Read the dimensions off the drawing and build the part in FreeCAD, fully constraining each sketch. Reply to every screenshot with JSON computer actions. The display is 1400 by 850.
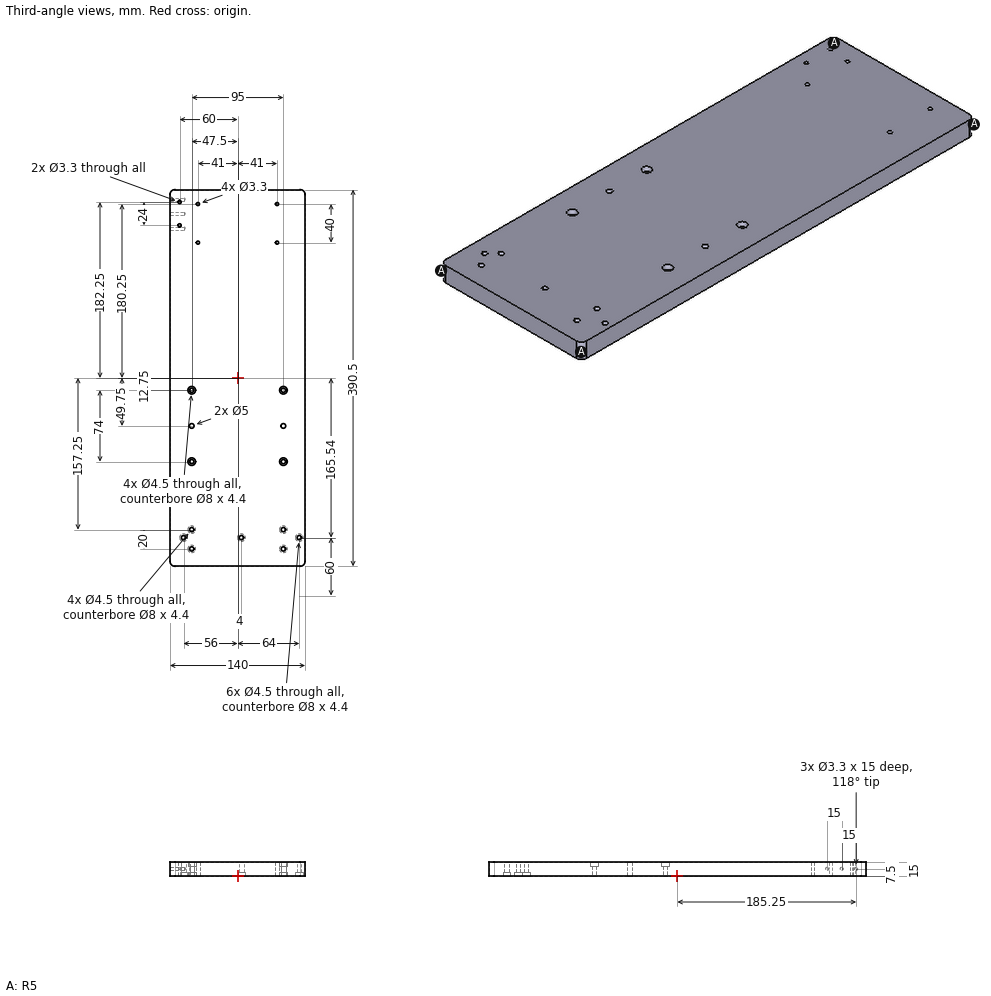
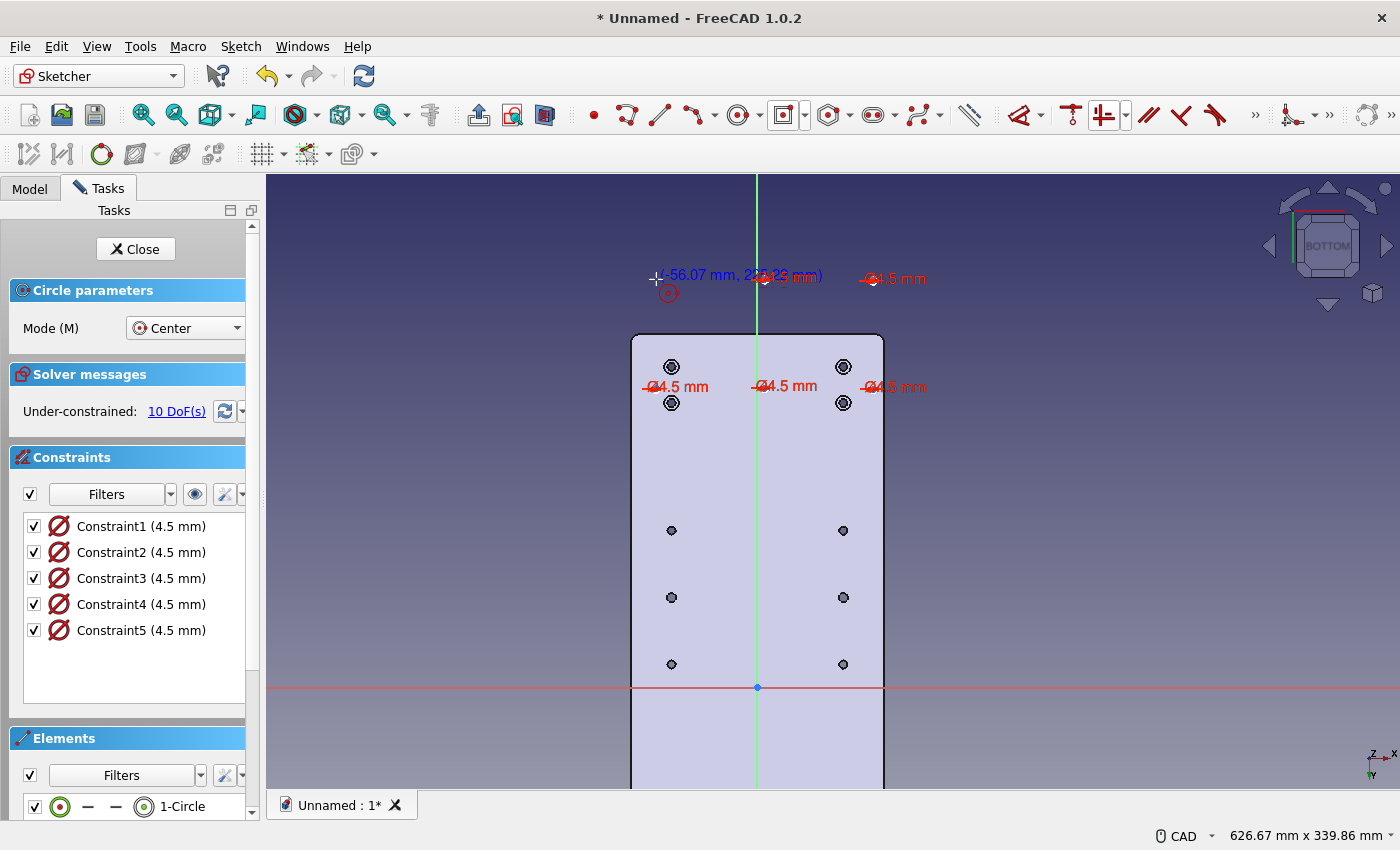
{"action": "left_click", "coordinate": [656, 279]}
{"action": "mouse_move", "coordinate": [659, 277]}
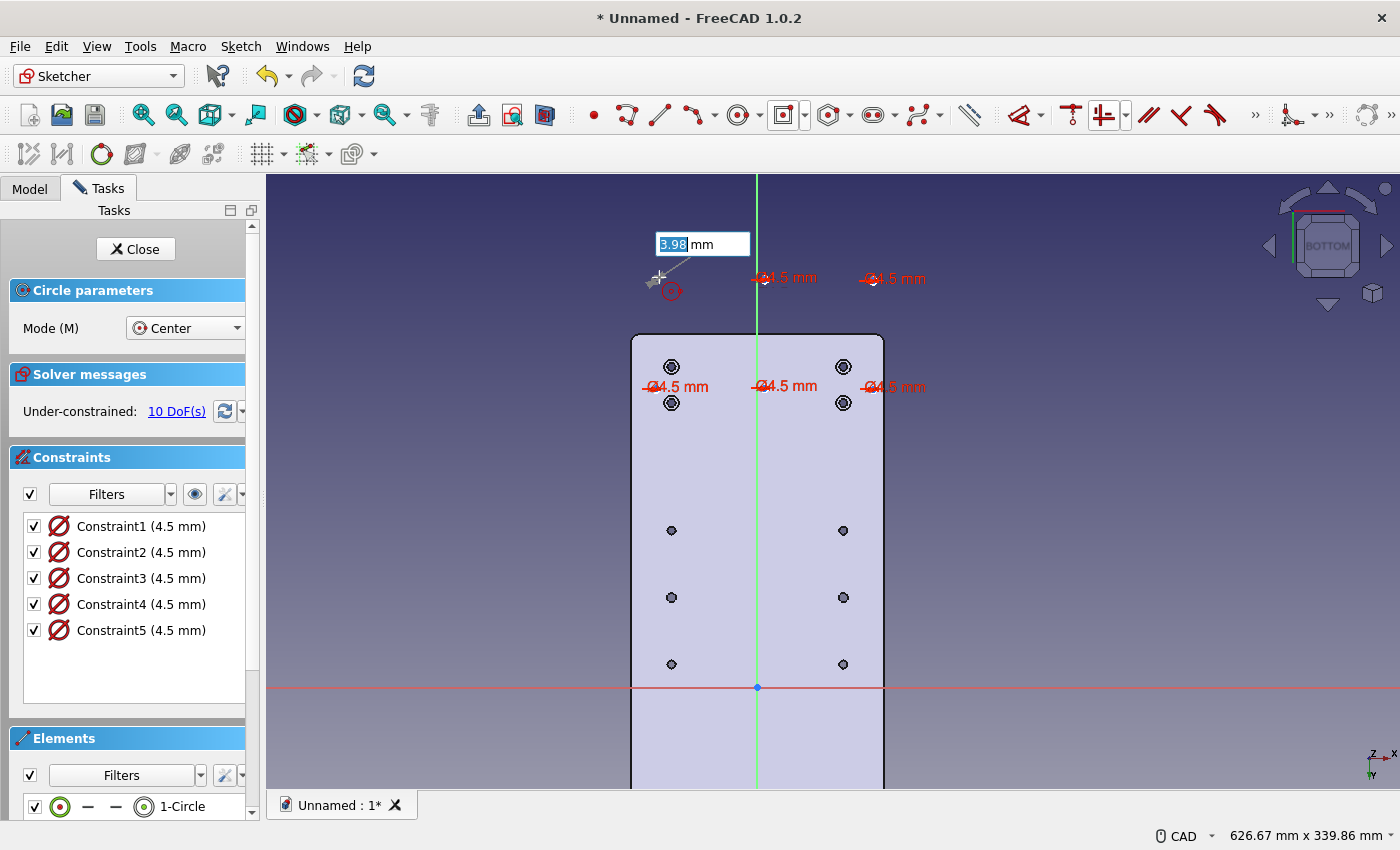
{"action": "type", "text": "4.5"}
{"action": "key", "text": "Return"}
{"action": "key", "text": "Escape"}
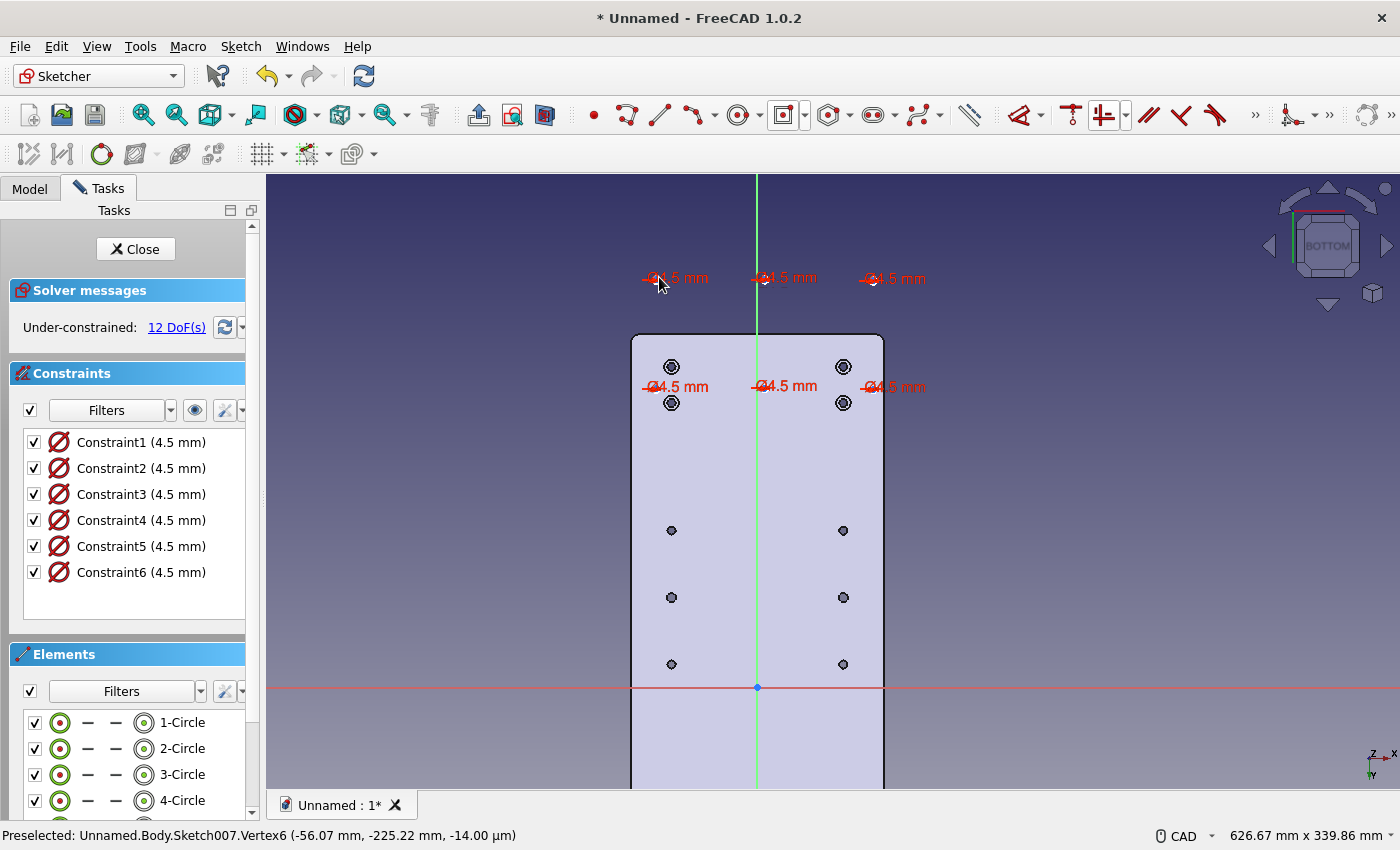
{"action": "left_click", "coordinate": [873, 389]}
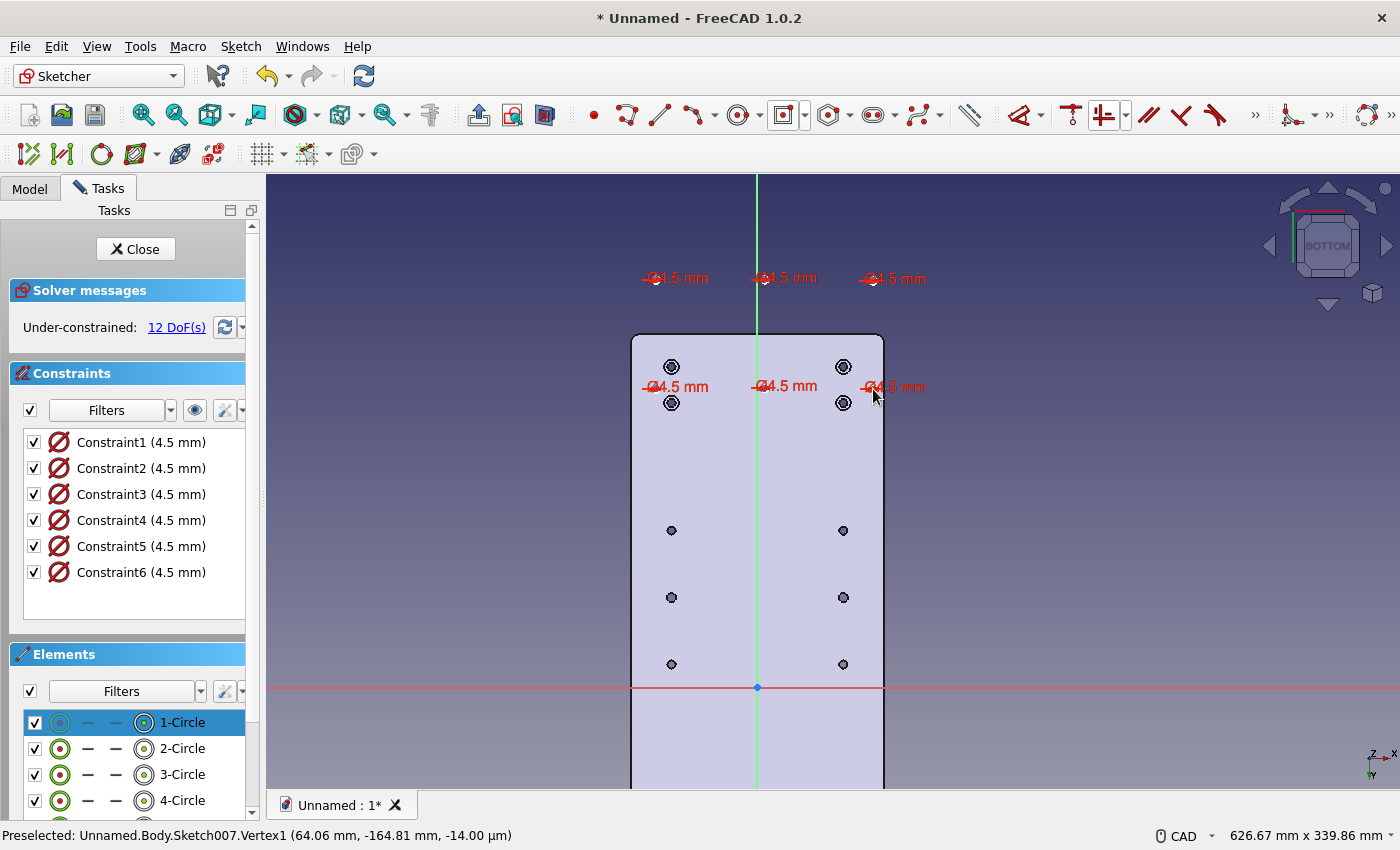
{"action": "left_click", "coordinate": [765, 388]}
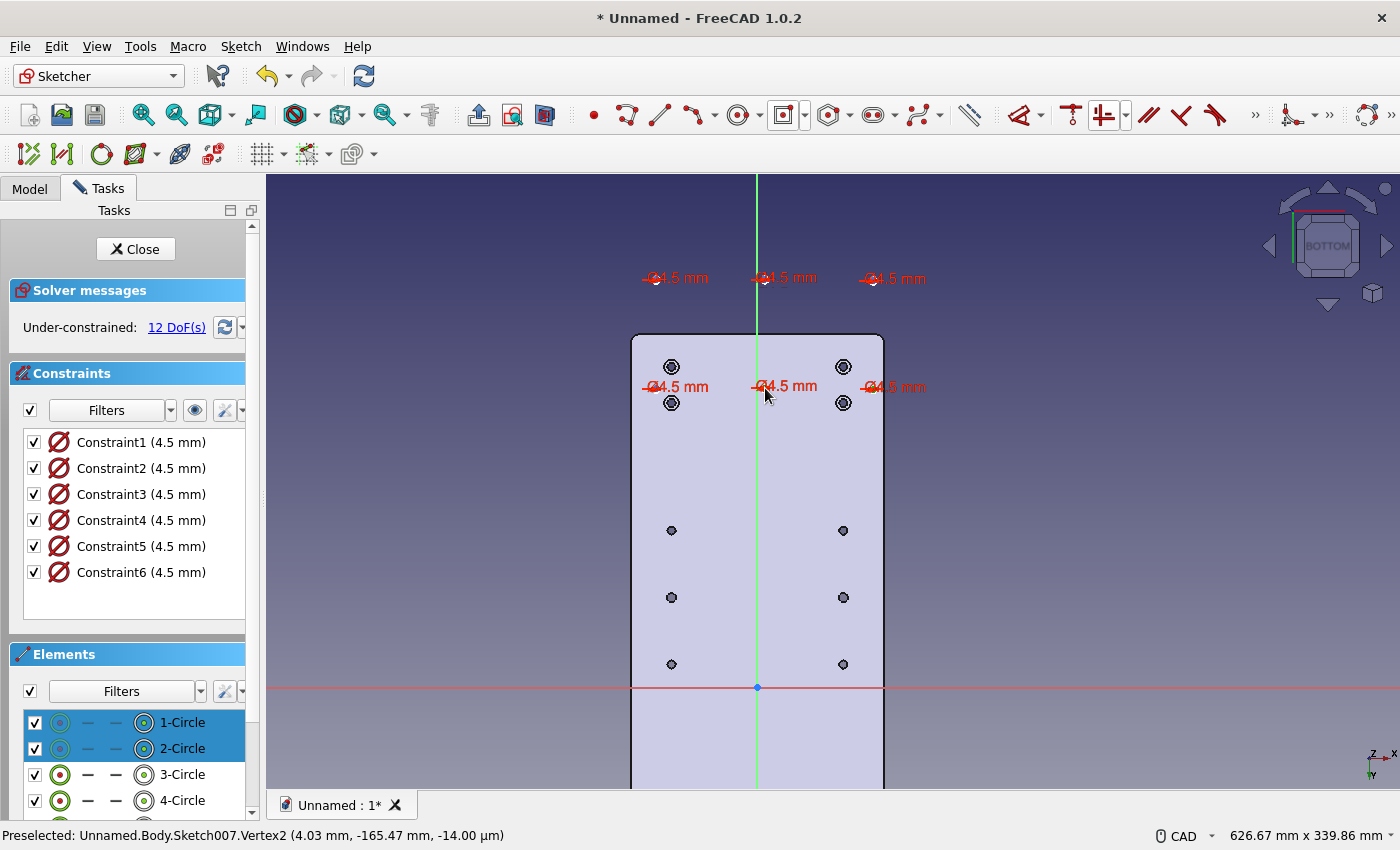
{"action": "key", "text": "h"}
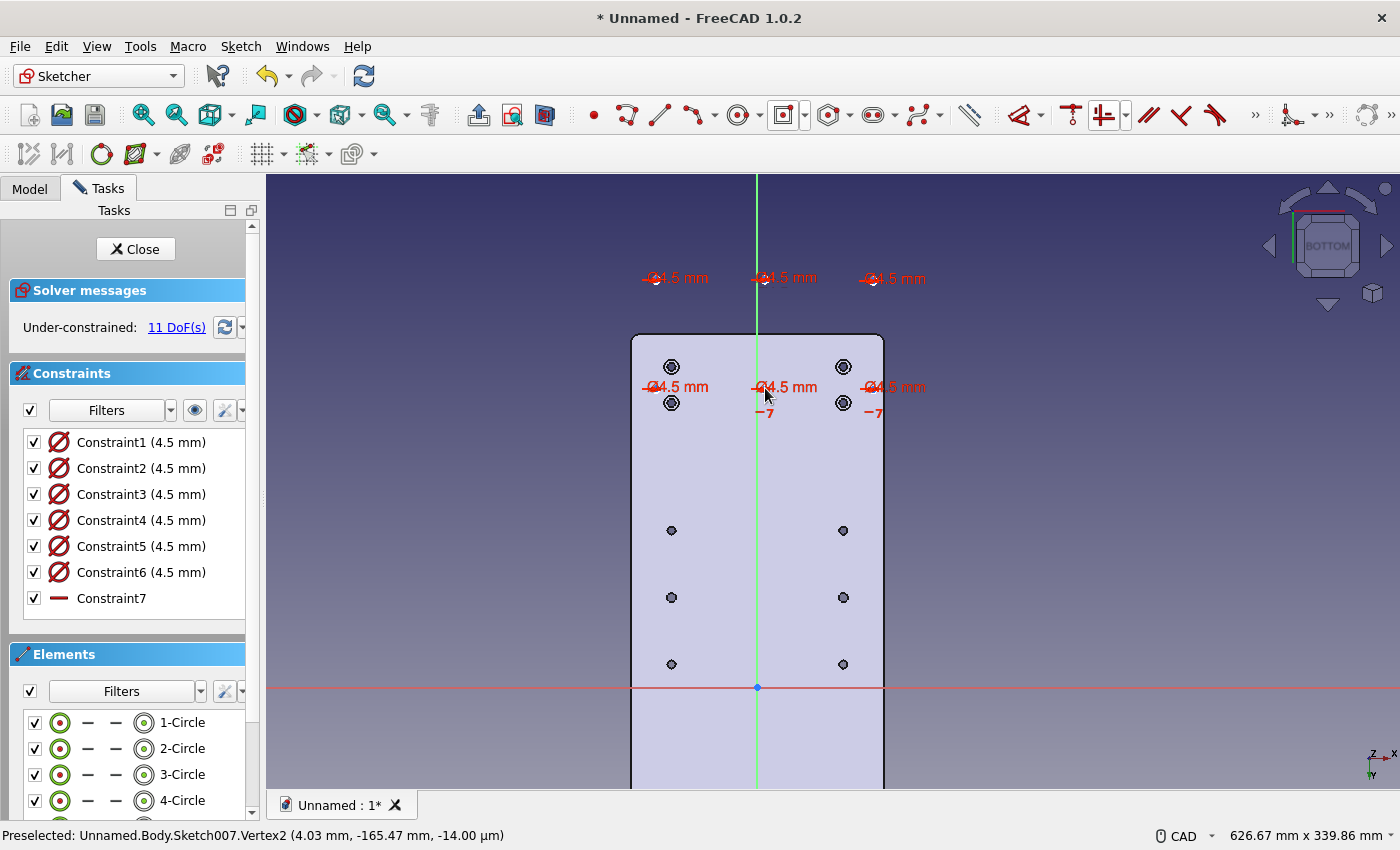
{"action": "left_click", "coordinate": [873, 389]}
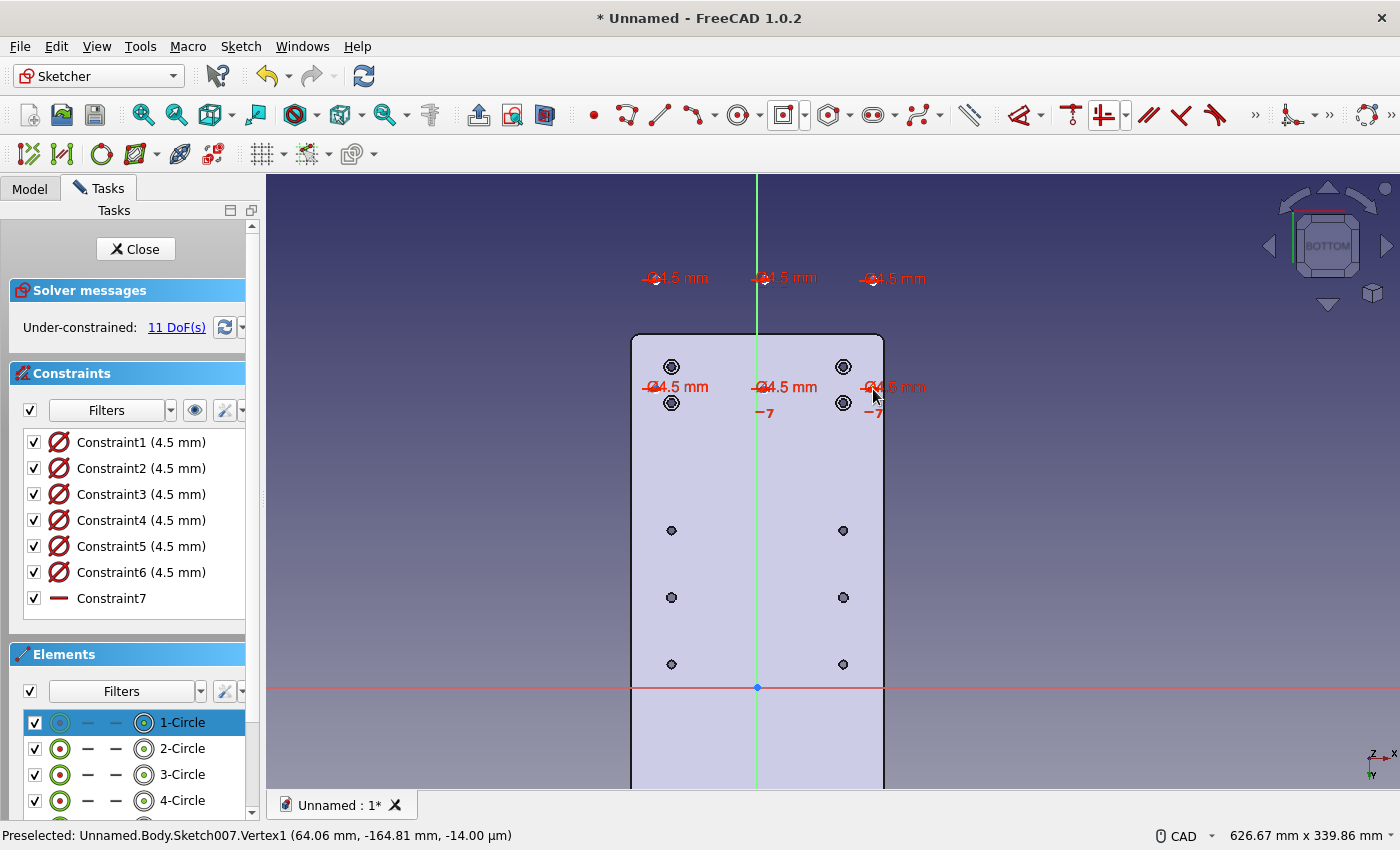
{"action": "left_click", "coordinate": [873, 281]}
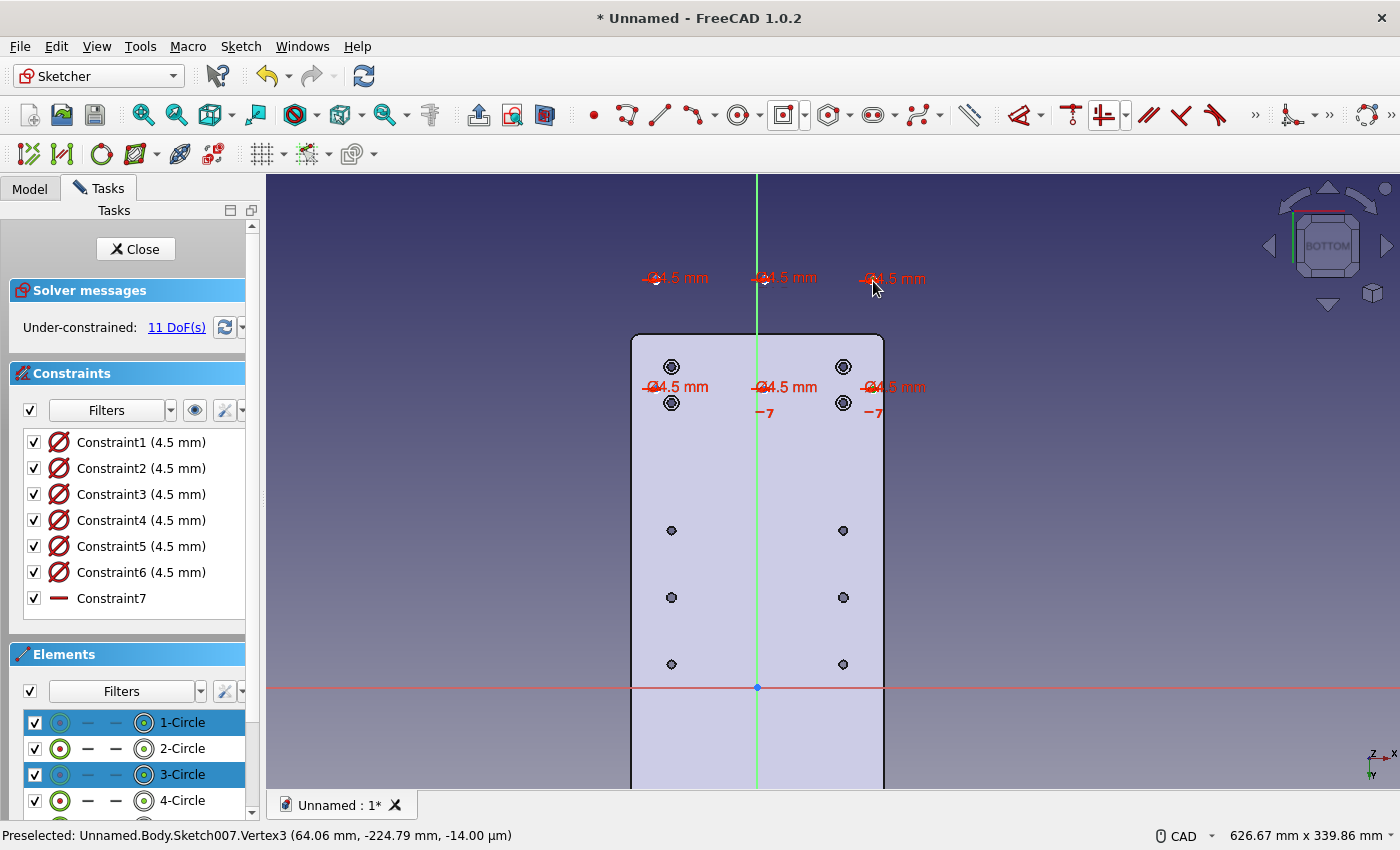
{"action": "key", "text": "v"}